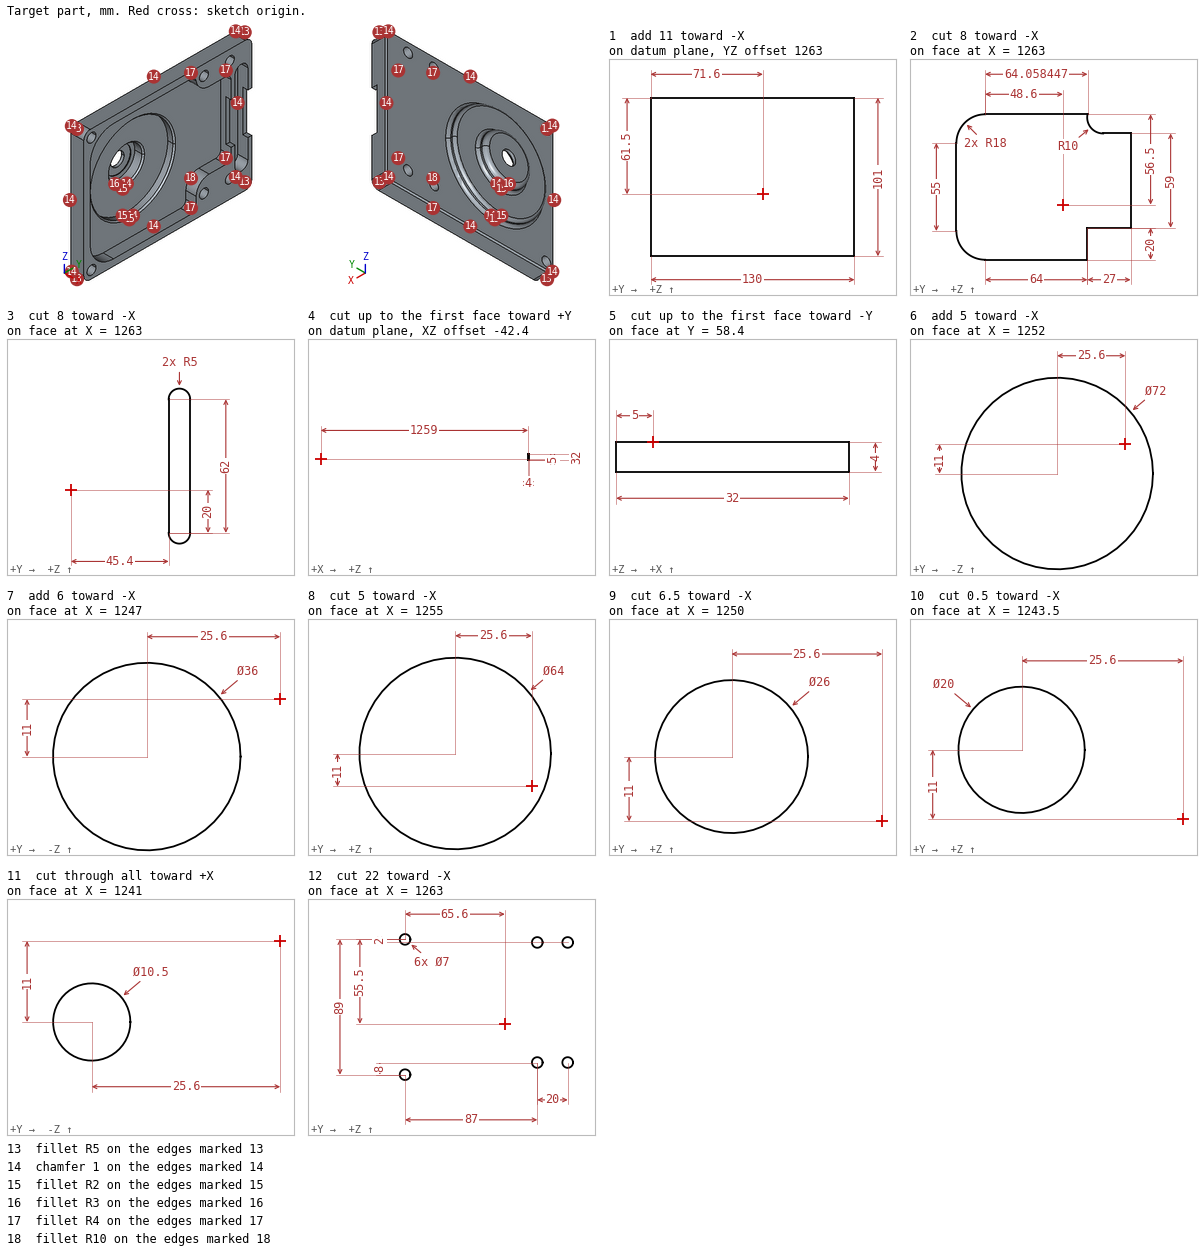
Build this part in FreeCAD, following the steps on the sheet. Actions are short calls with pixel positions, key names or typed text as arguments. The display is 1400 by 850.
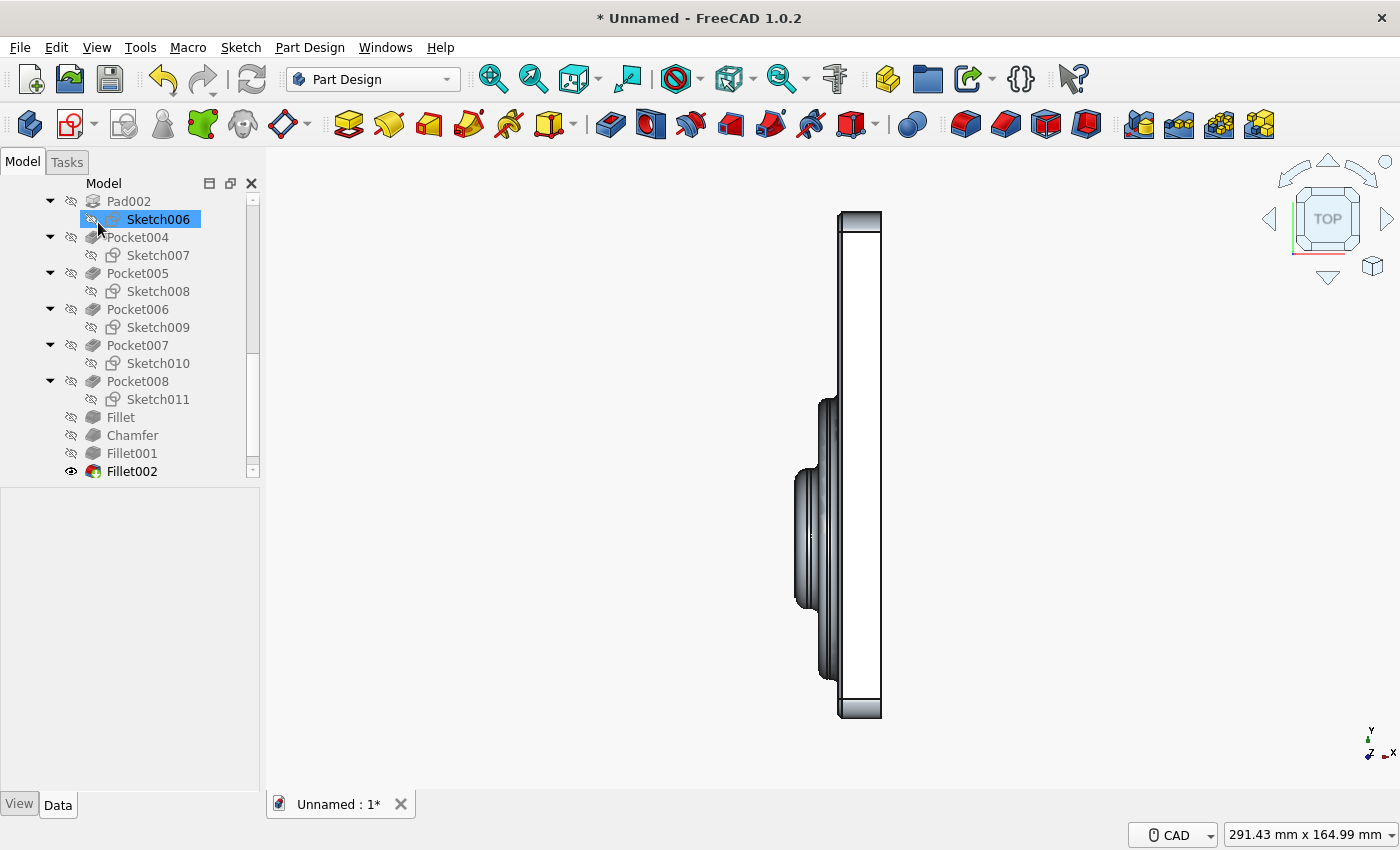
key(1)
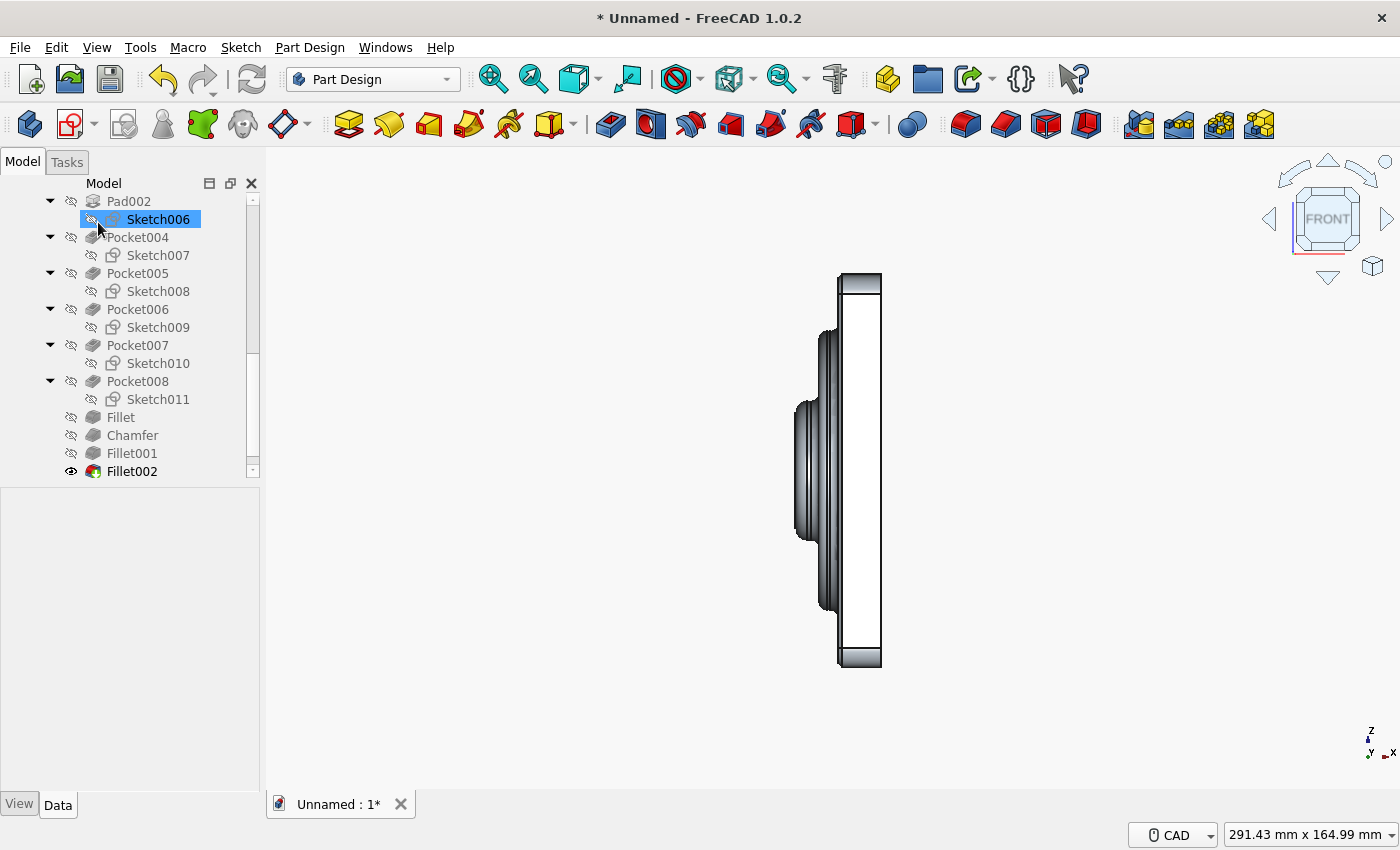
key(3)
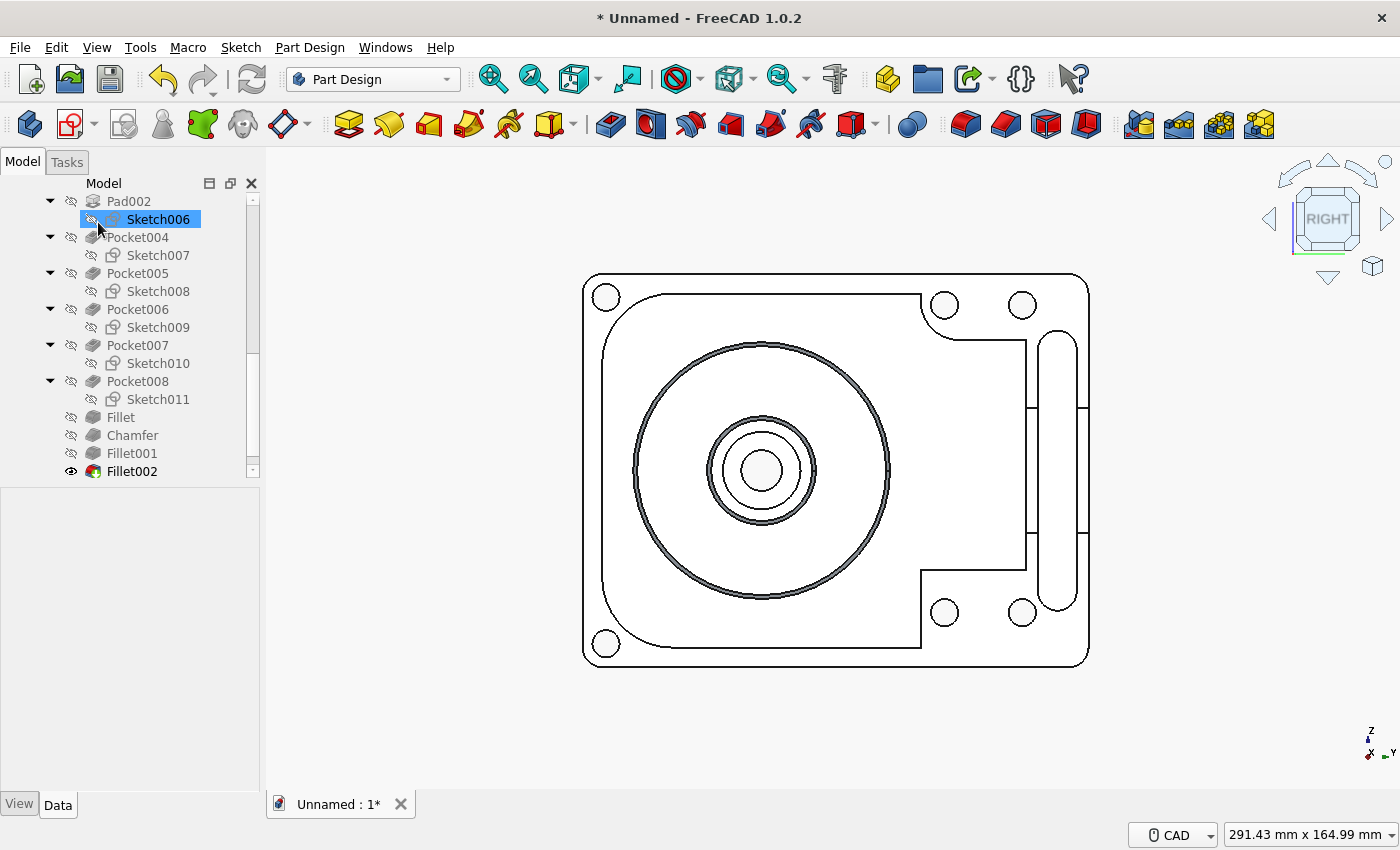
key(5)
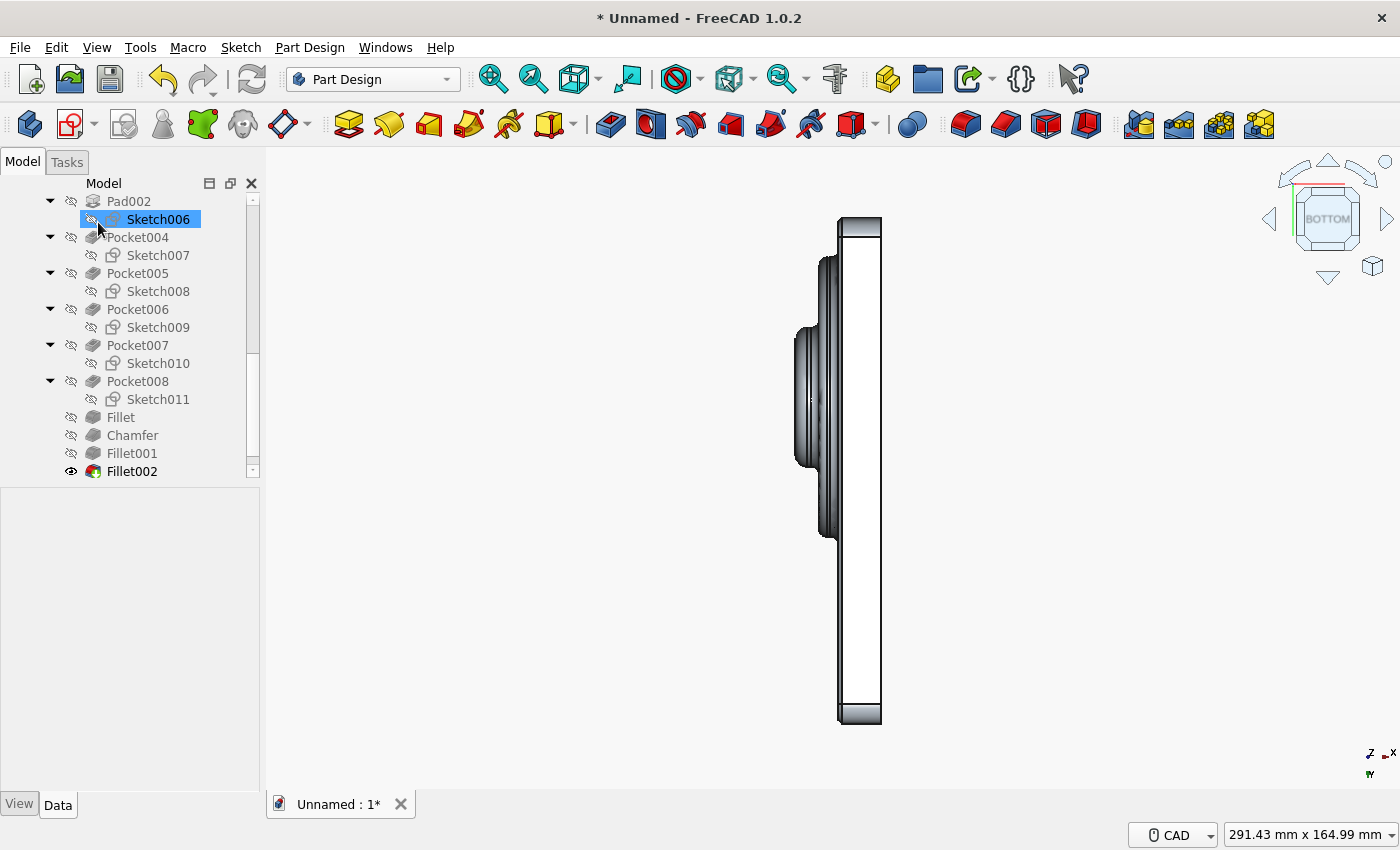
key(4)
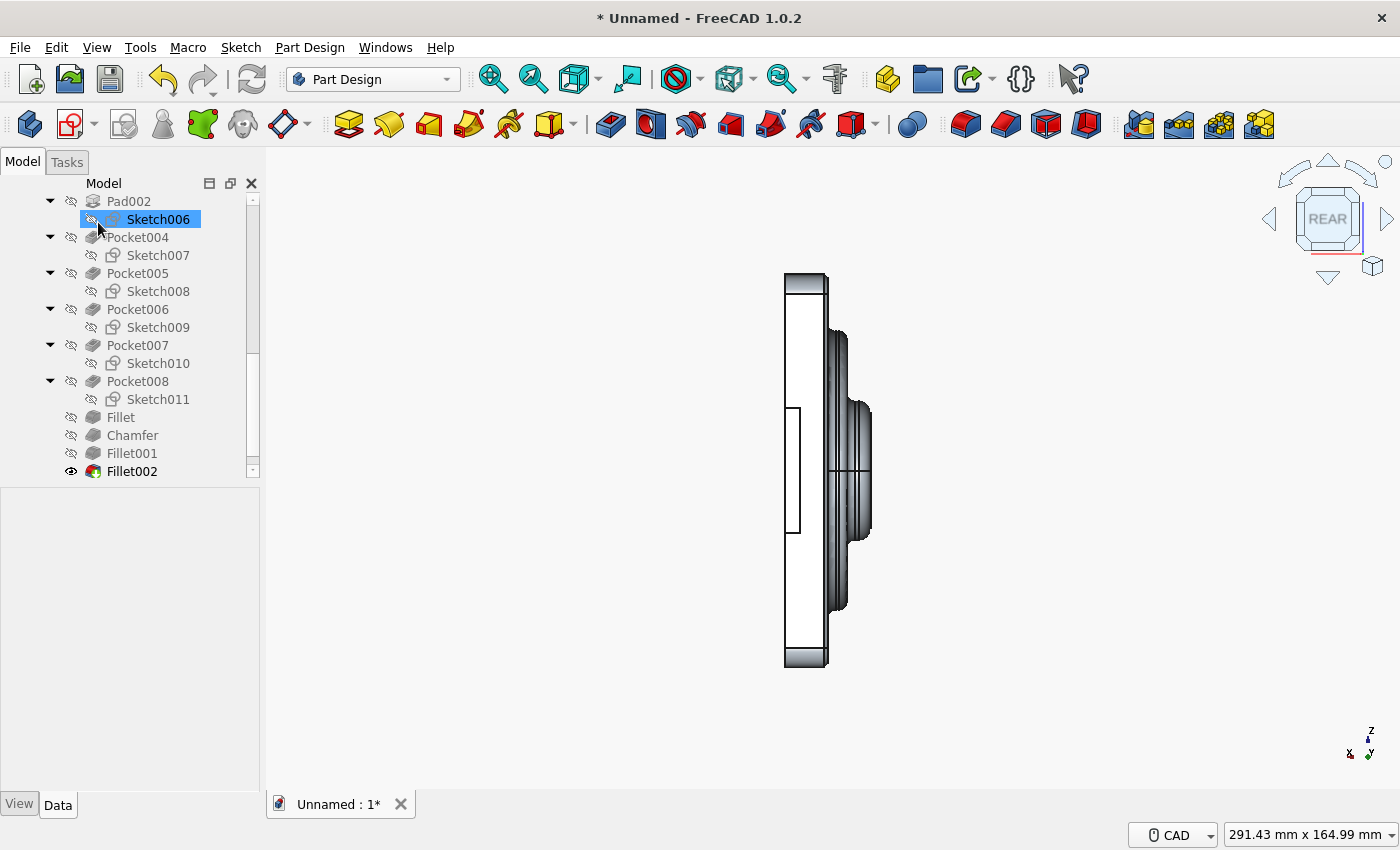
key(6)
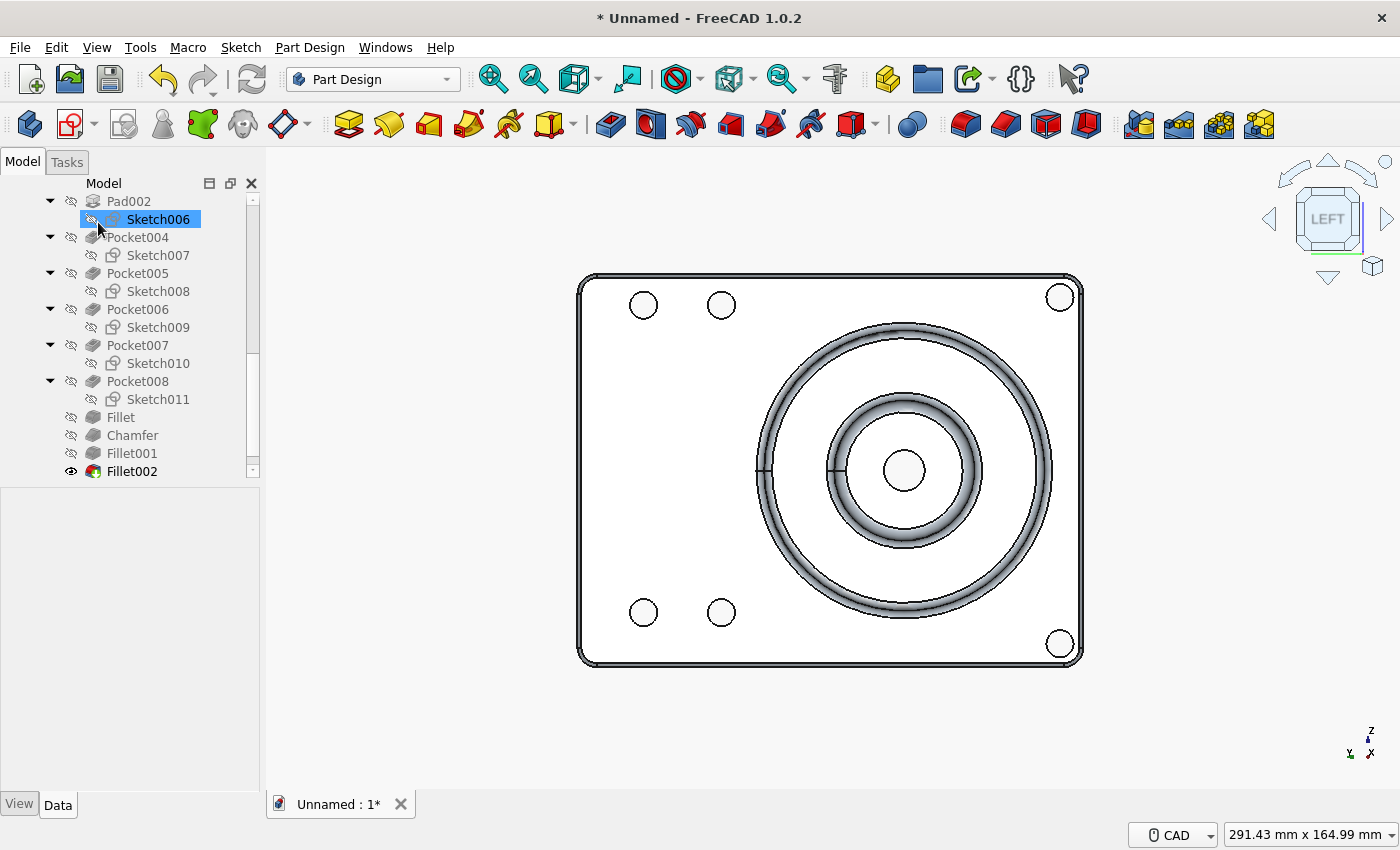
key(v)
key(3)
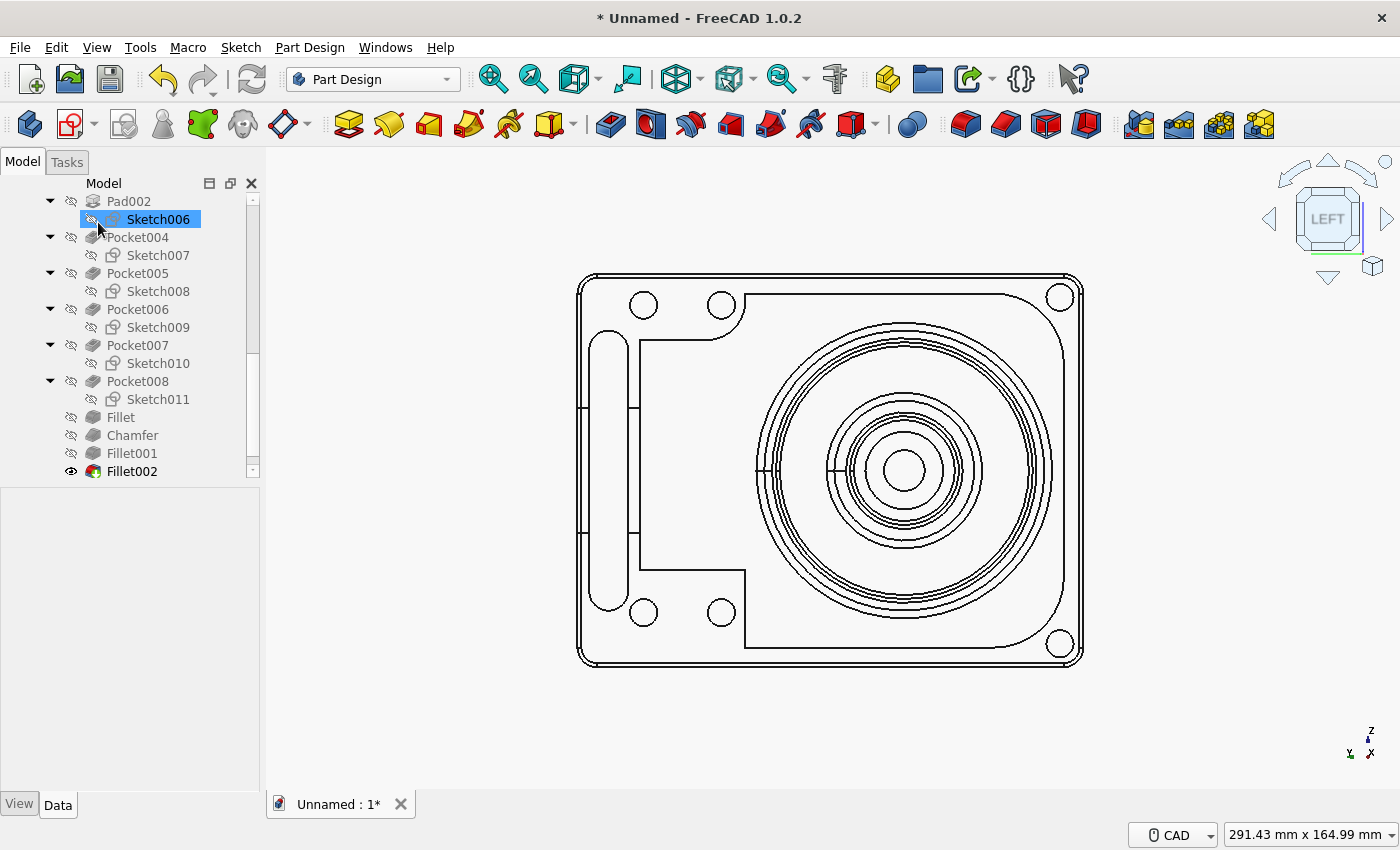
key(0)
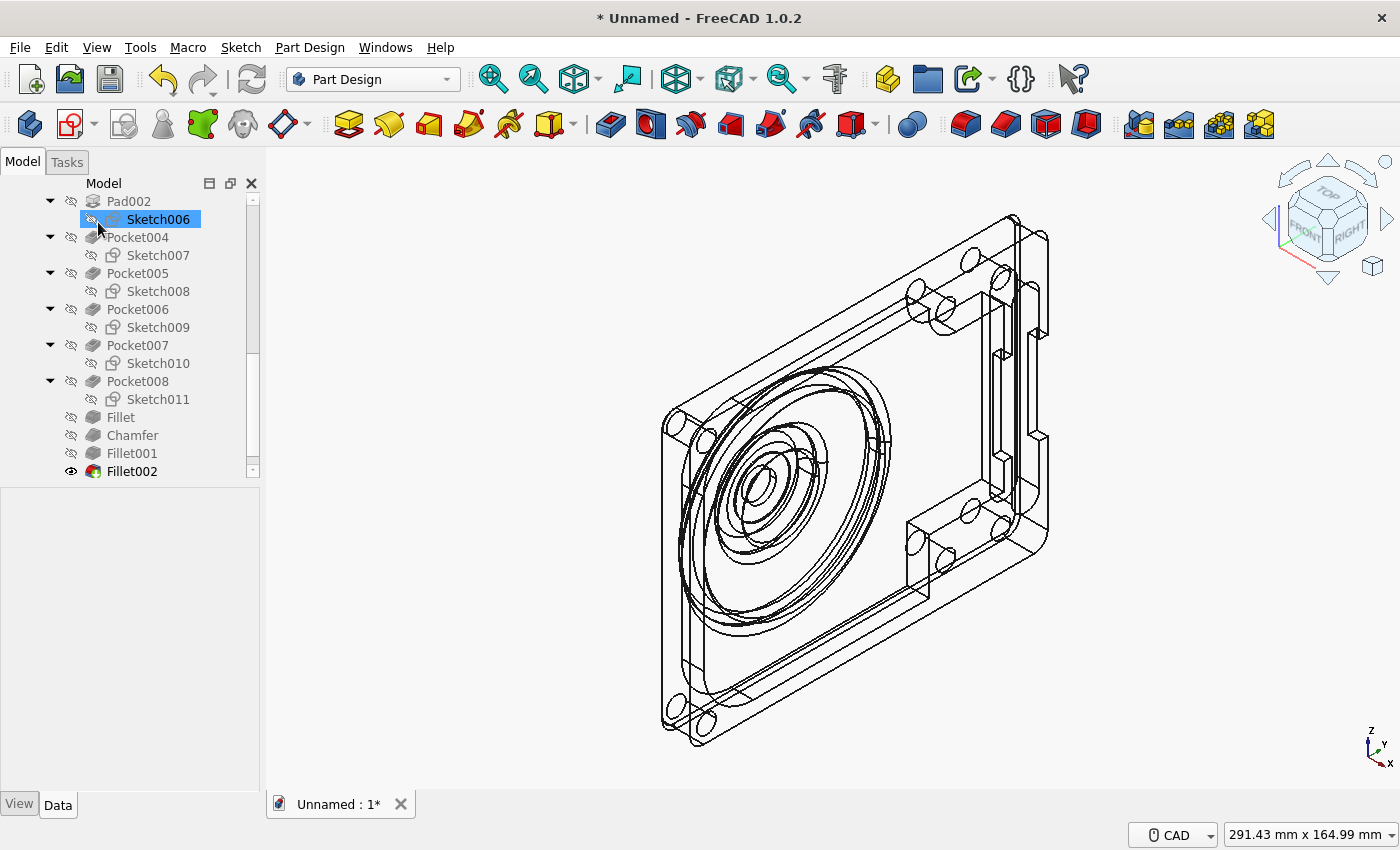
click(993, 485)